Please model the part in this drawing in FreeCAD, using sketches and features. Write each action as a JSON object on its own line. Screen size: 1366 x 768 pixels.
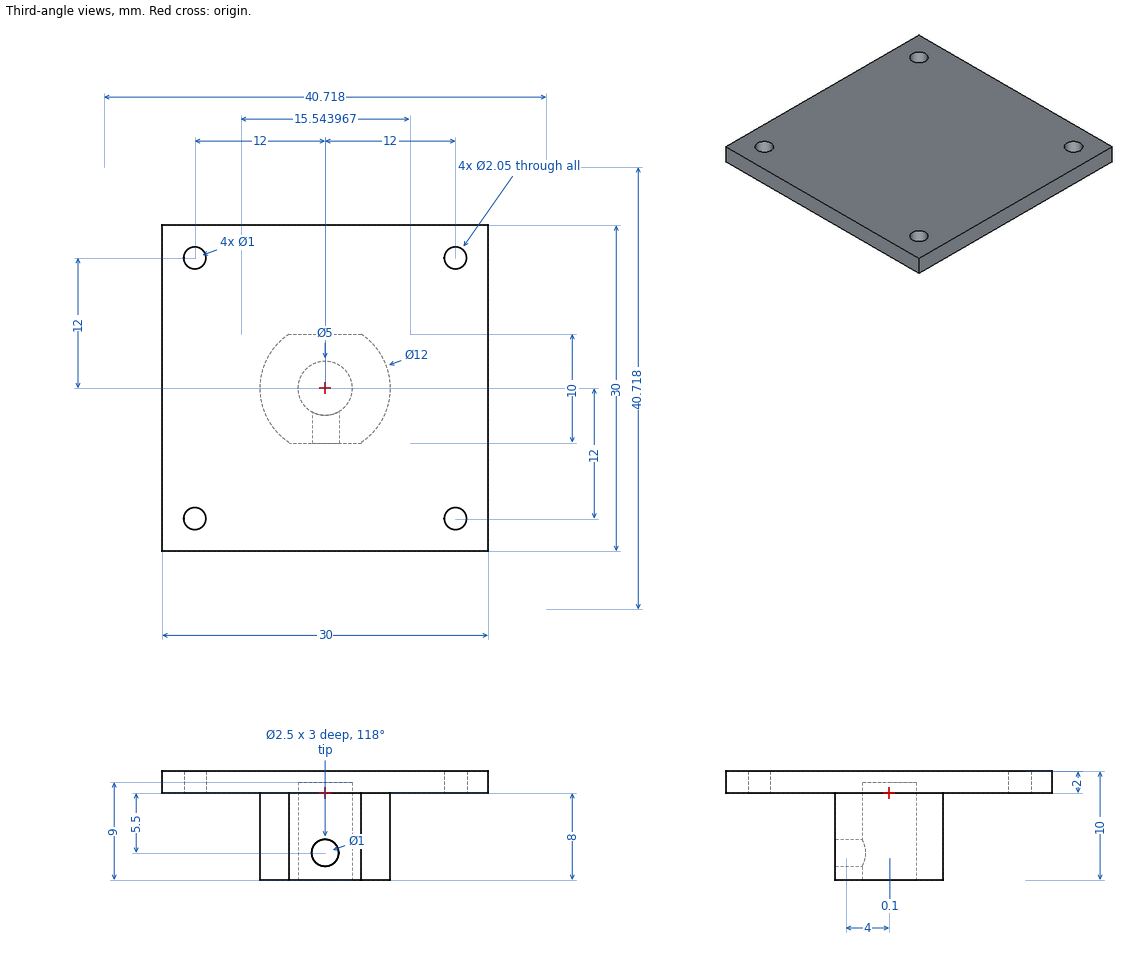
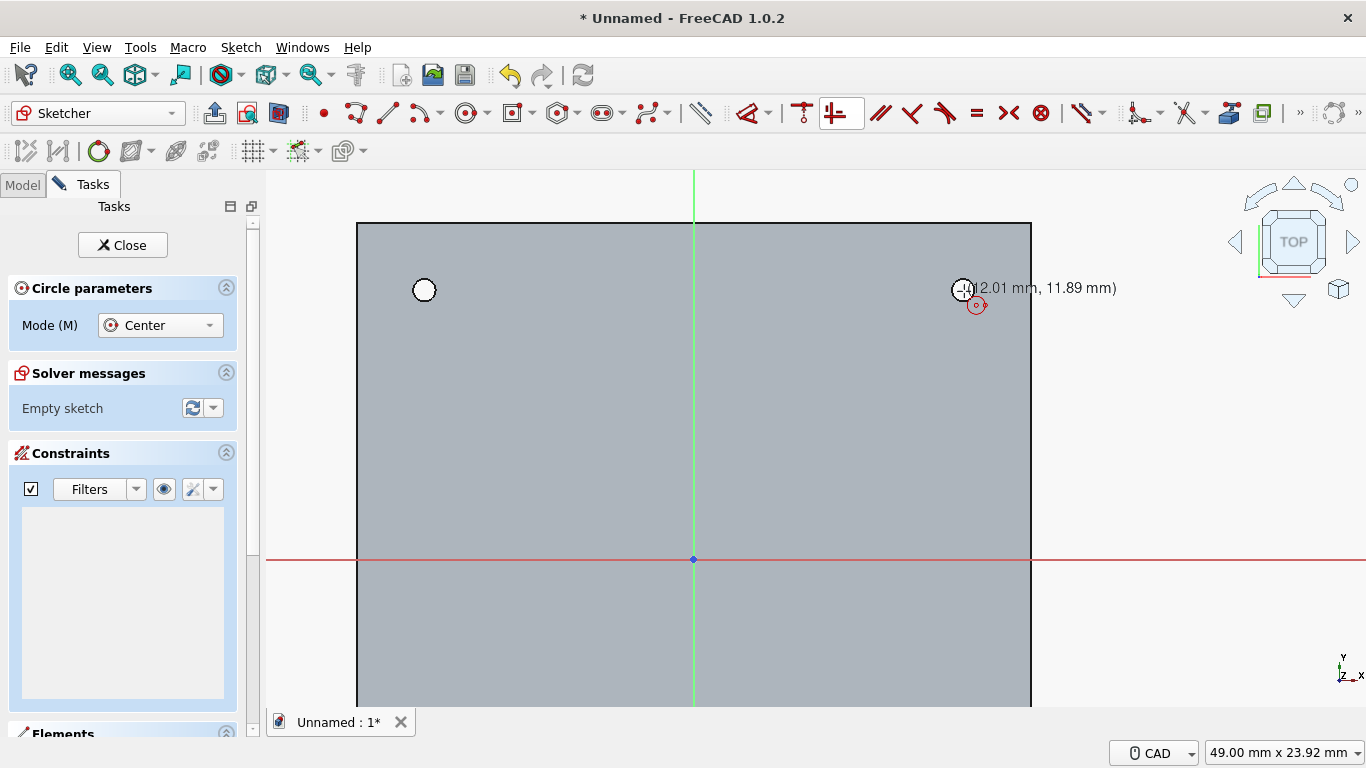
{"action": "left_click", "coordinate": [963, 290]}
{"action": "left_click", "coordinate": [979, 274]}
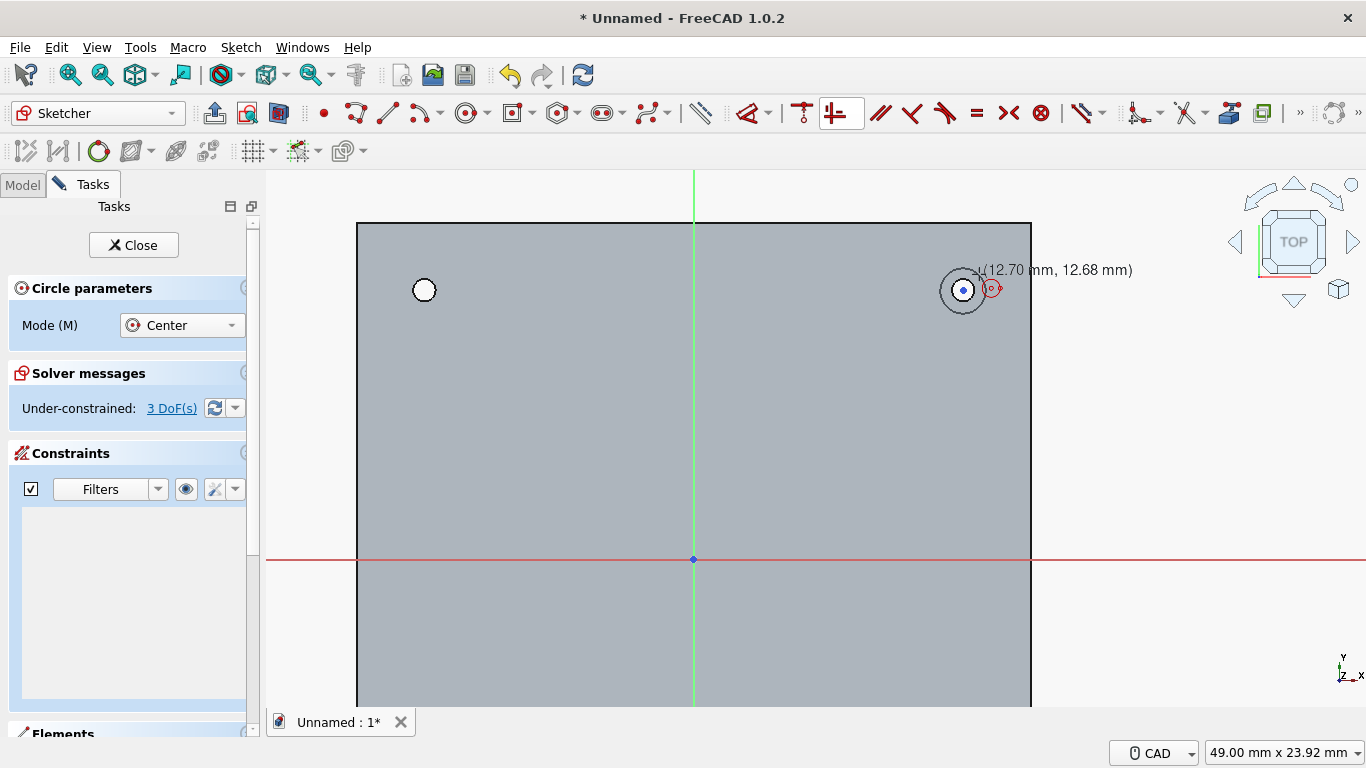
{"action": "scroll", "coordinate": [813, 291], "scroll_direction": "down", "scroll_amount": 3}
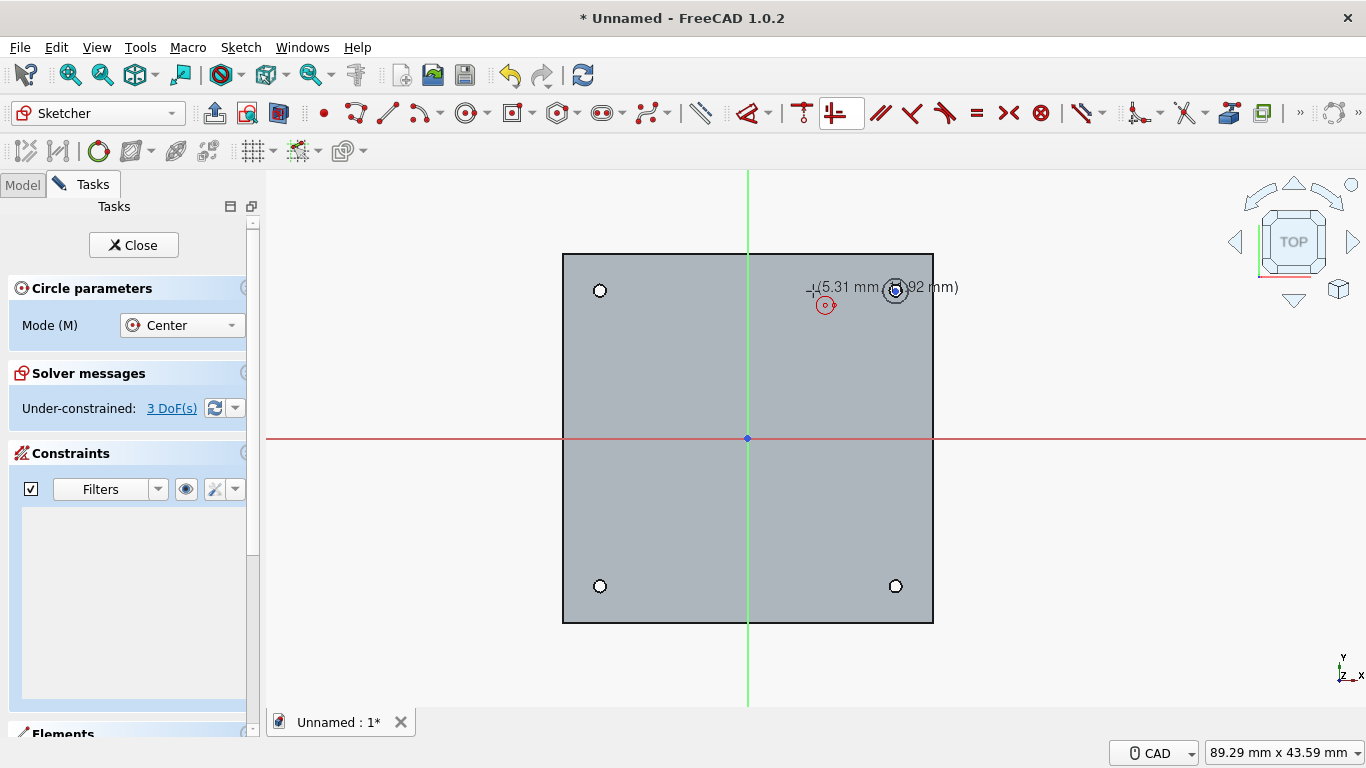
{"action": "scroll", "coordinate": [896, 586], "scroll_direction": "up", "scroll_amount": 3}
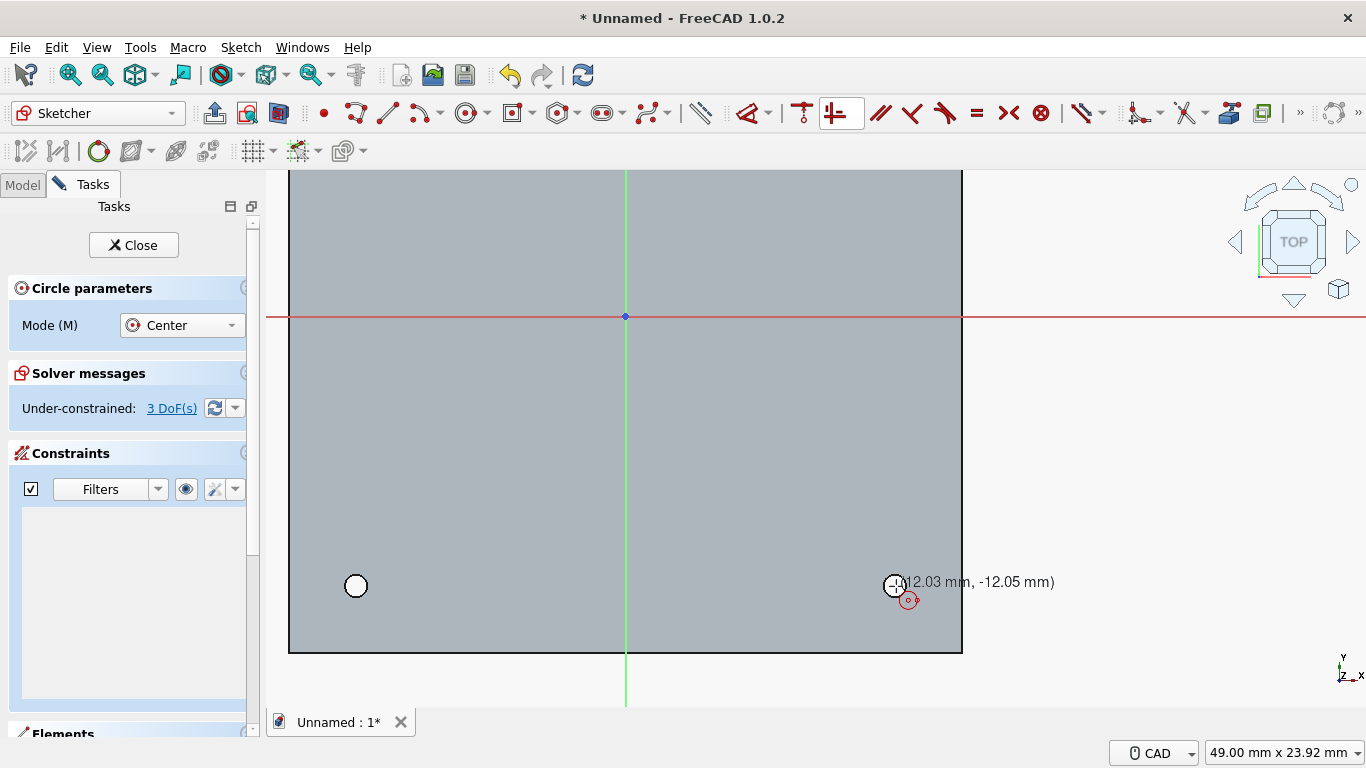
{"action": "left_click", "coordinate": [895, 586]}
{"action": "left_click", "coordinate": [911, 570]}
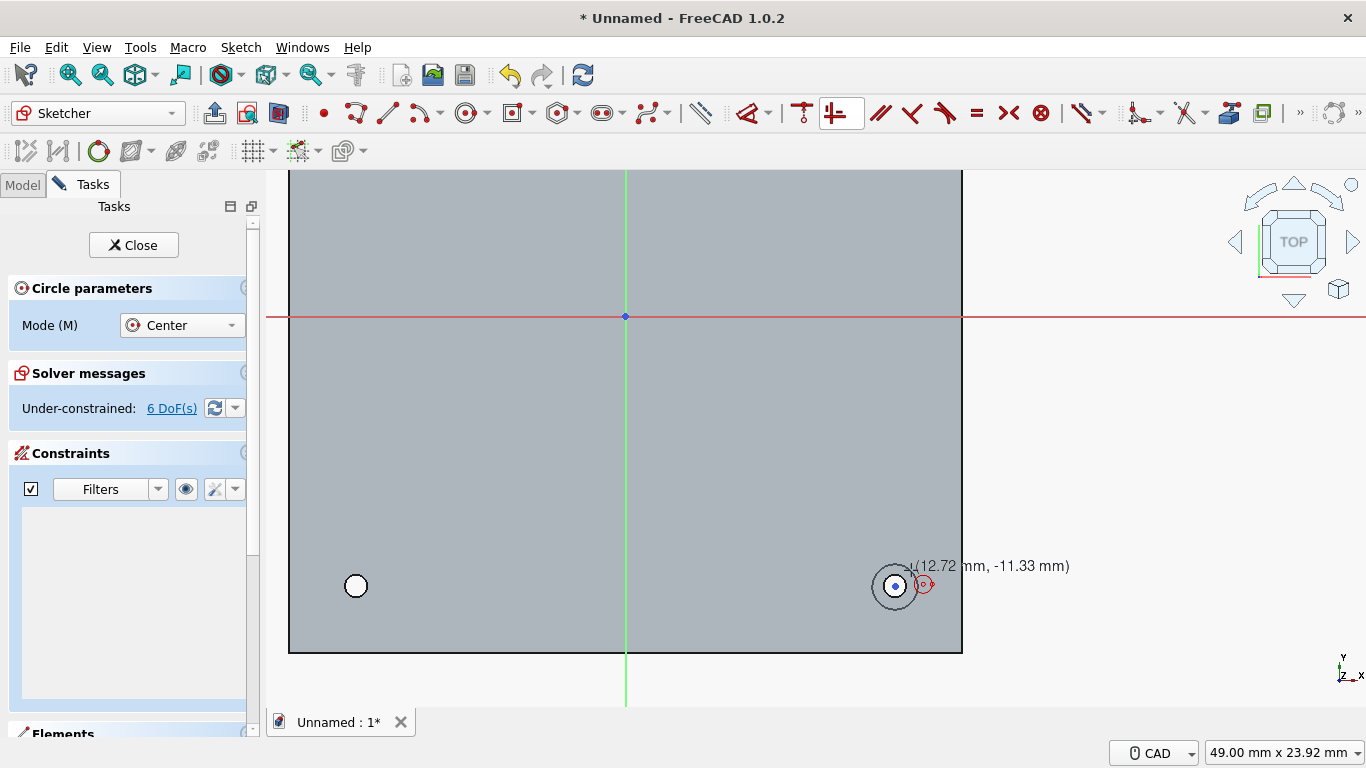
{"action": "left_click", "coordinate": [356, 586]}
{"action": "left_click", "coordinate": [372, 570]}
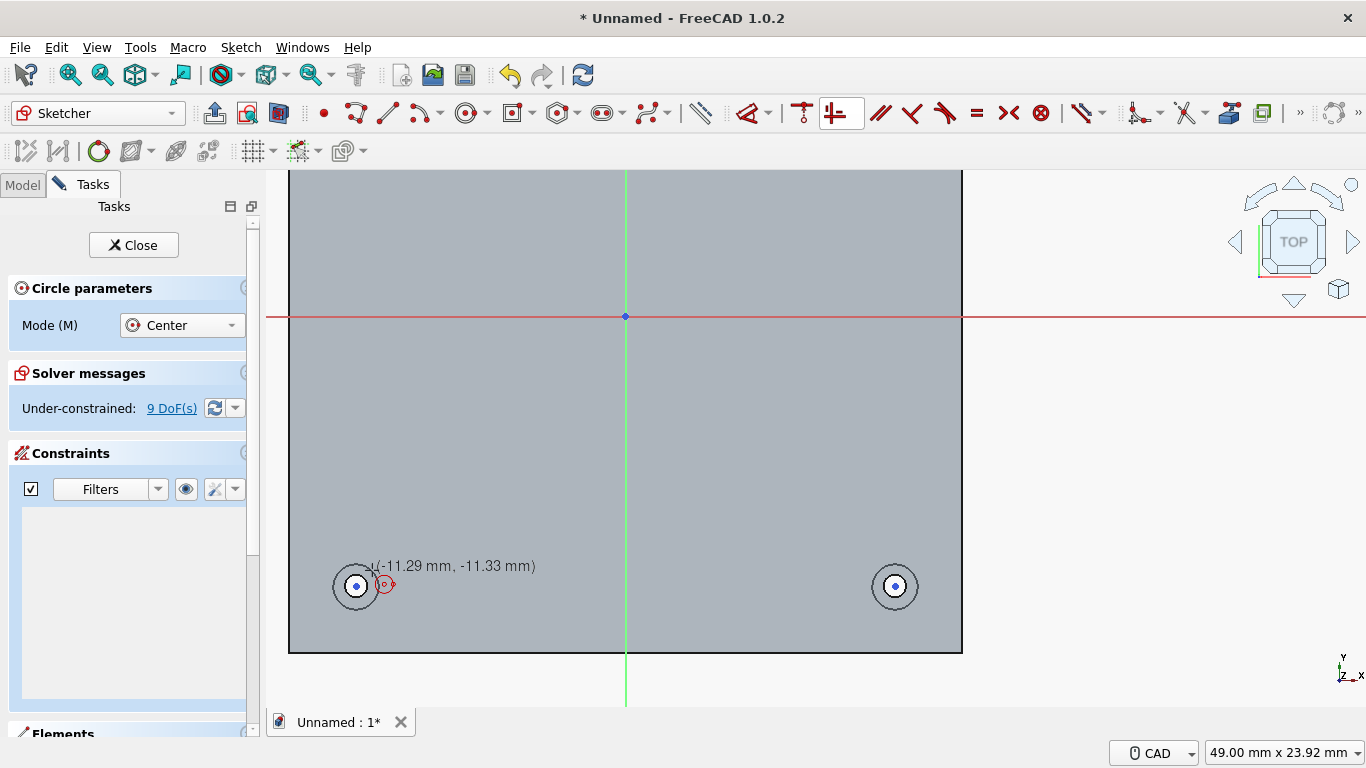
{"action": "scroll", "coordinate": [896, 587], "scroll_direction": "down", "scroll_amount": 3}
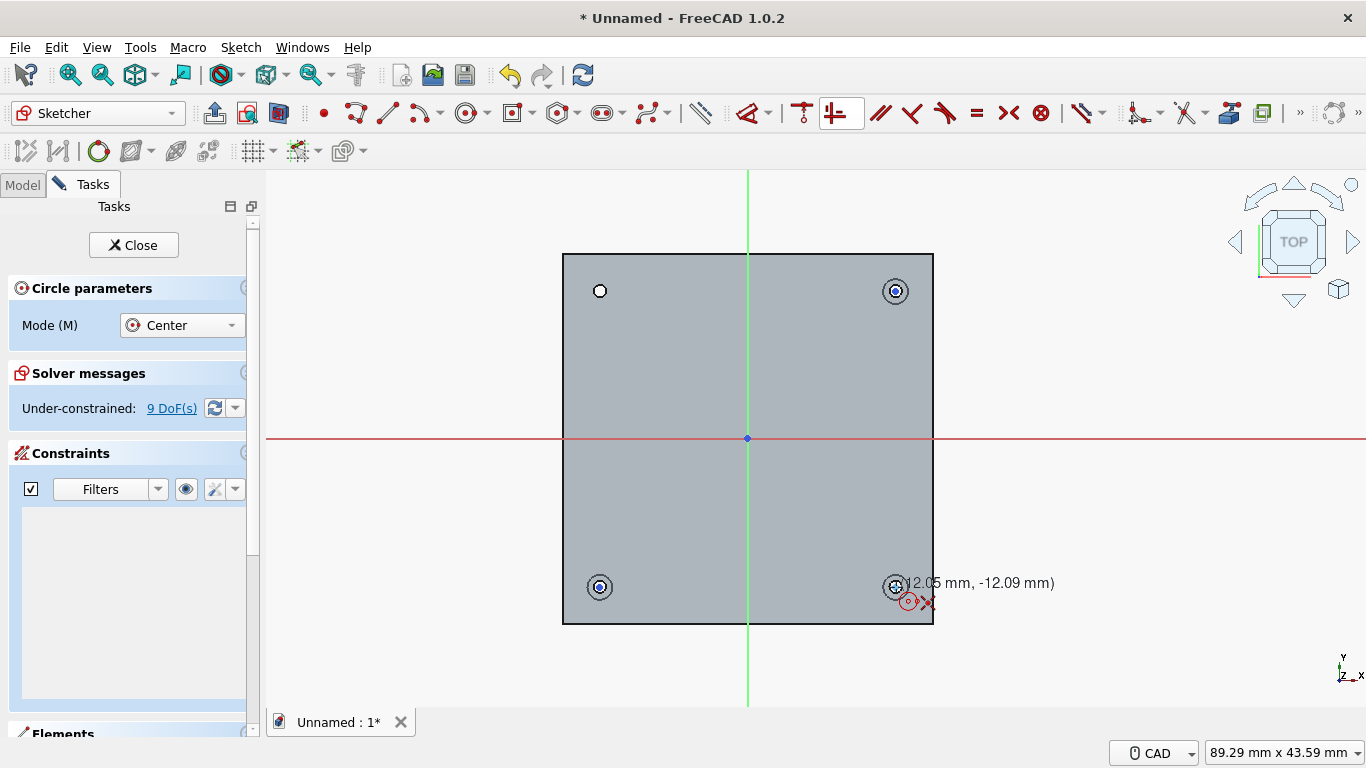
{"action": "scroll", "coordinate": [600, 291], "scroll_direction": "up", "scroll_amount": 3}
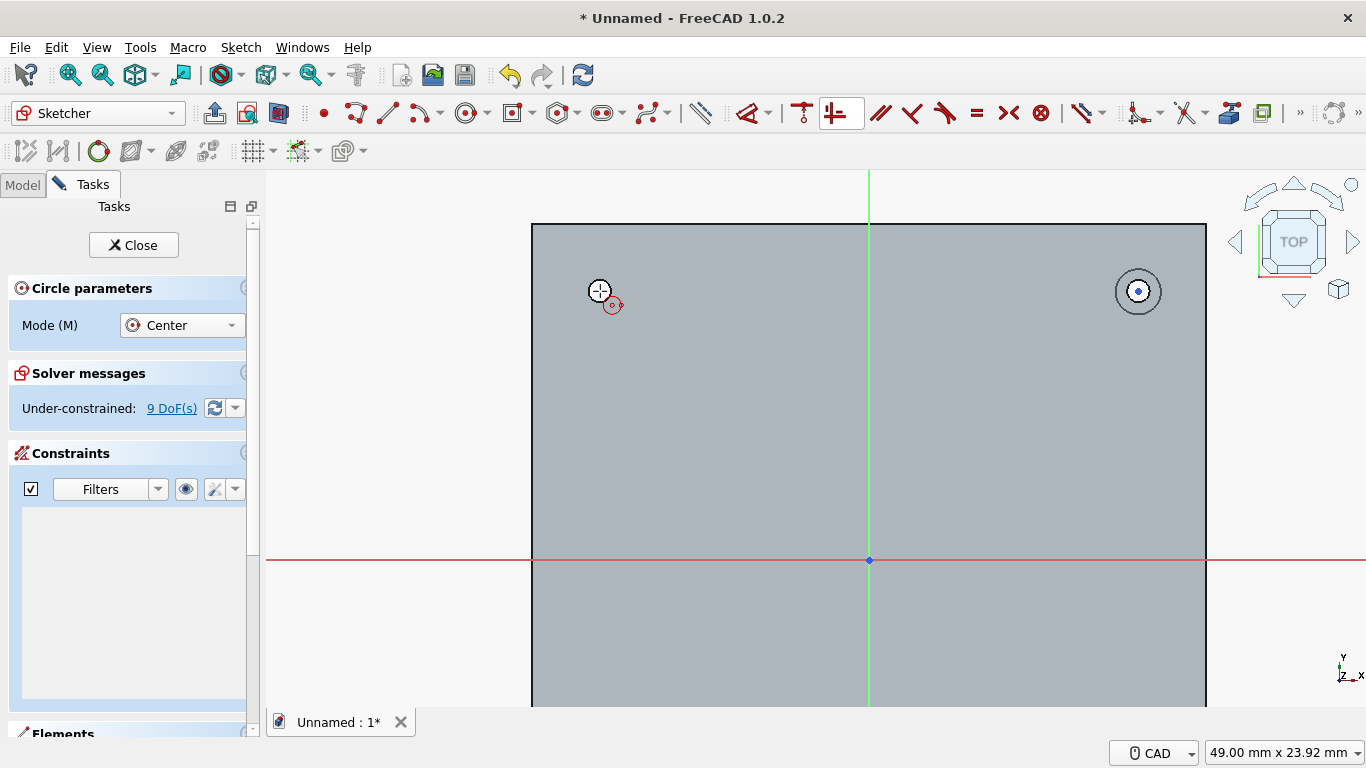
{"action": "left_click", "coordinate": [600, 291]}
{"action": "left_click", "coordinate": [616, 275]}
{"action": "key", "text": "Escape"}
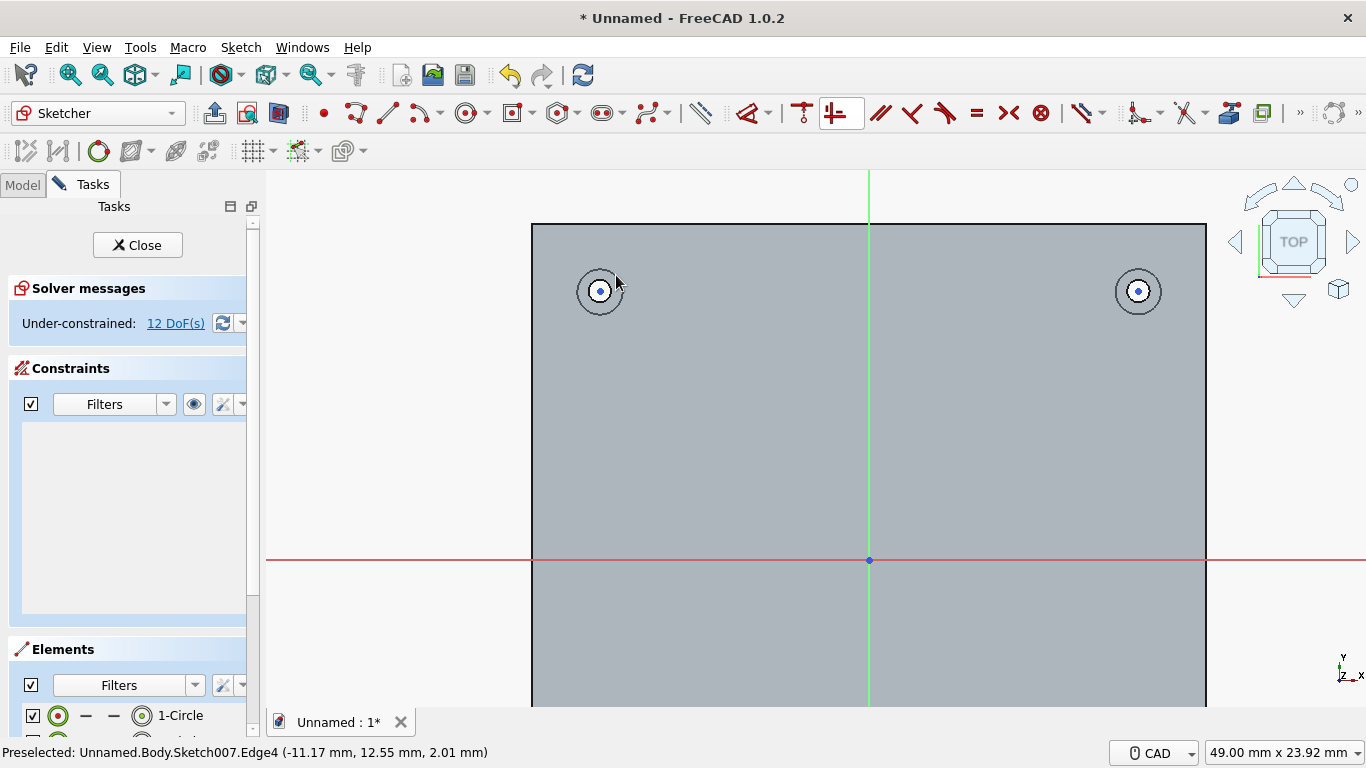
{"action": "left_click", "coordinate": [1154, 276]}